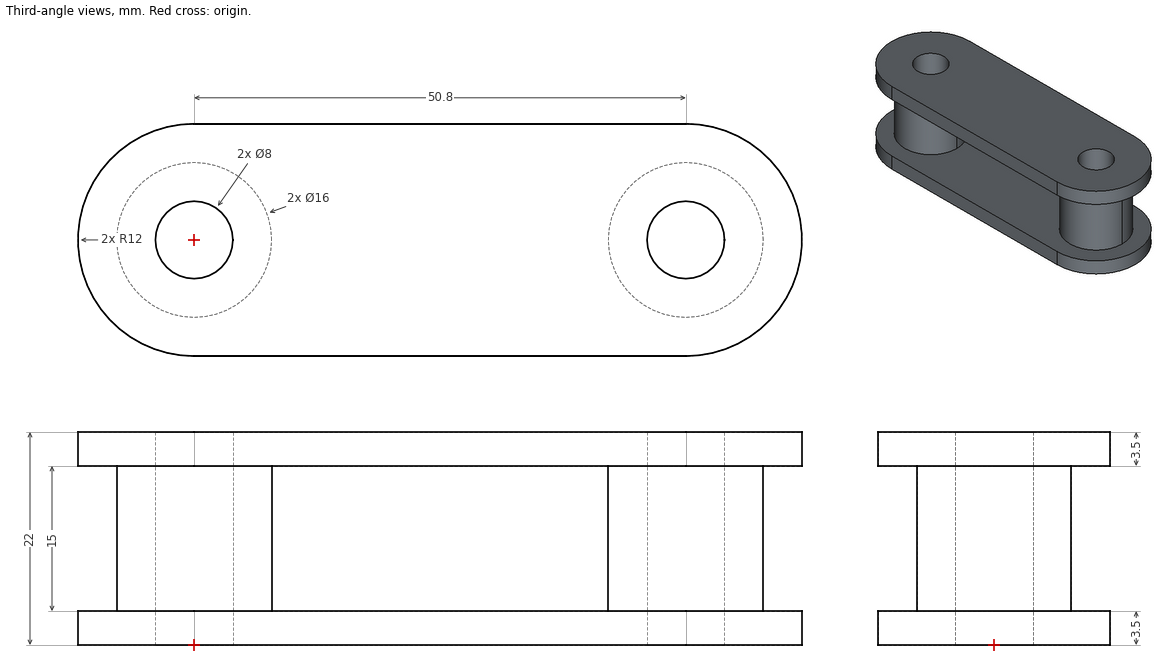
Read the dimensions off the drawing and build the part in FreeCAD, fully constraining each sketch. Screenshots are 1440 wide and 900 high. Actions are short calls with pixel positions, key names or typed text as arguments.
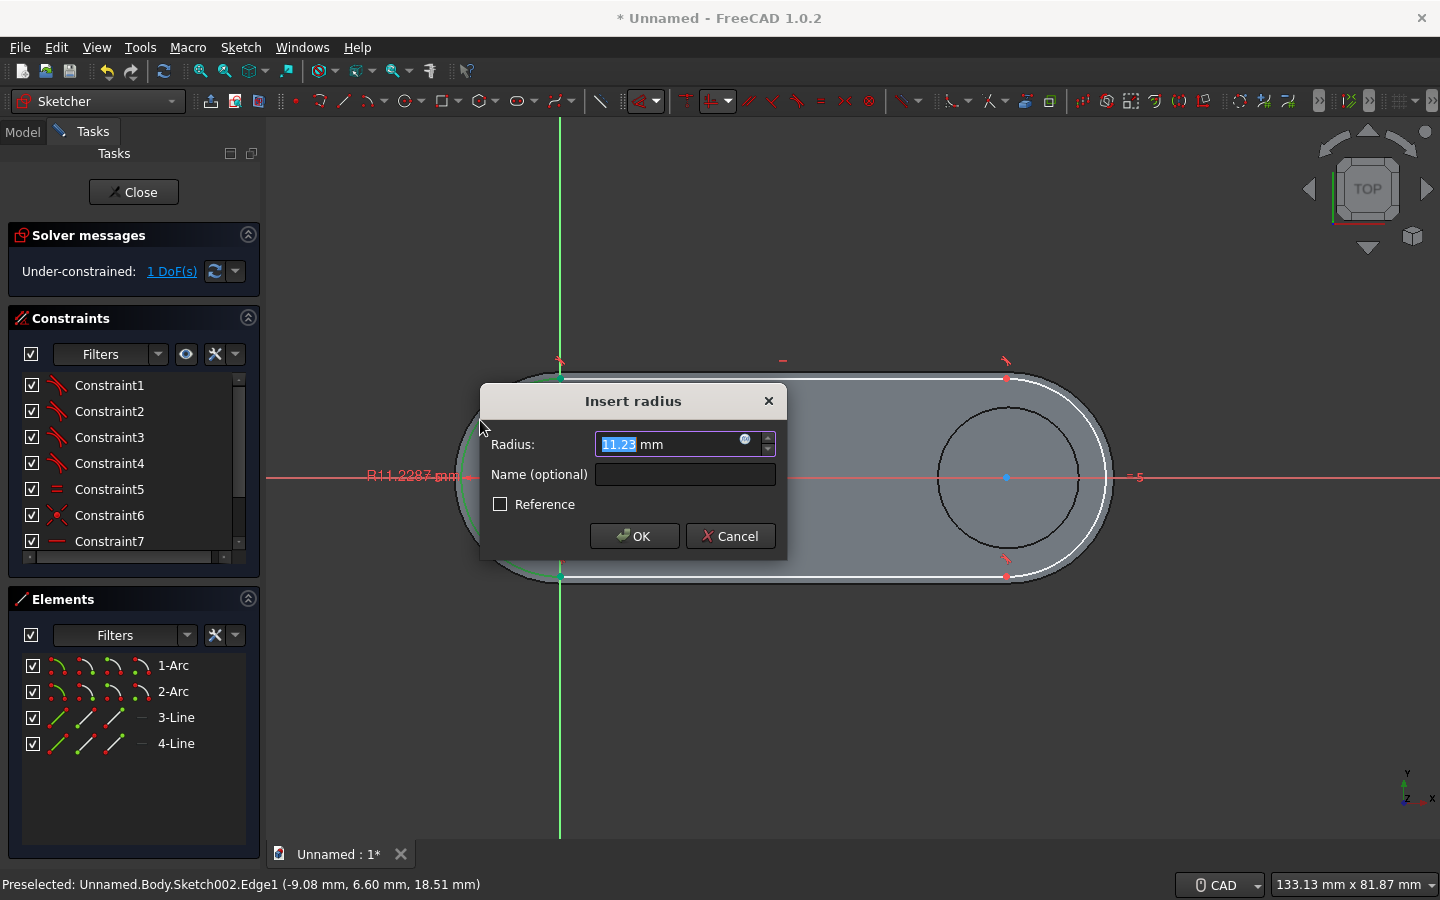
text(12)
key(Return)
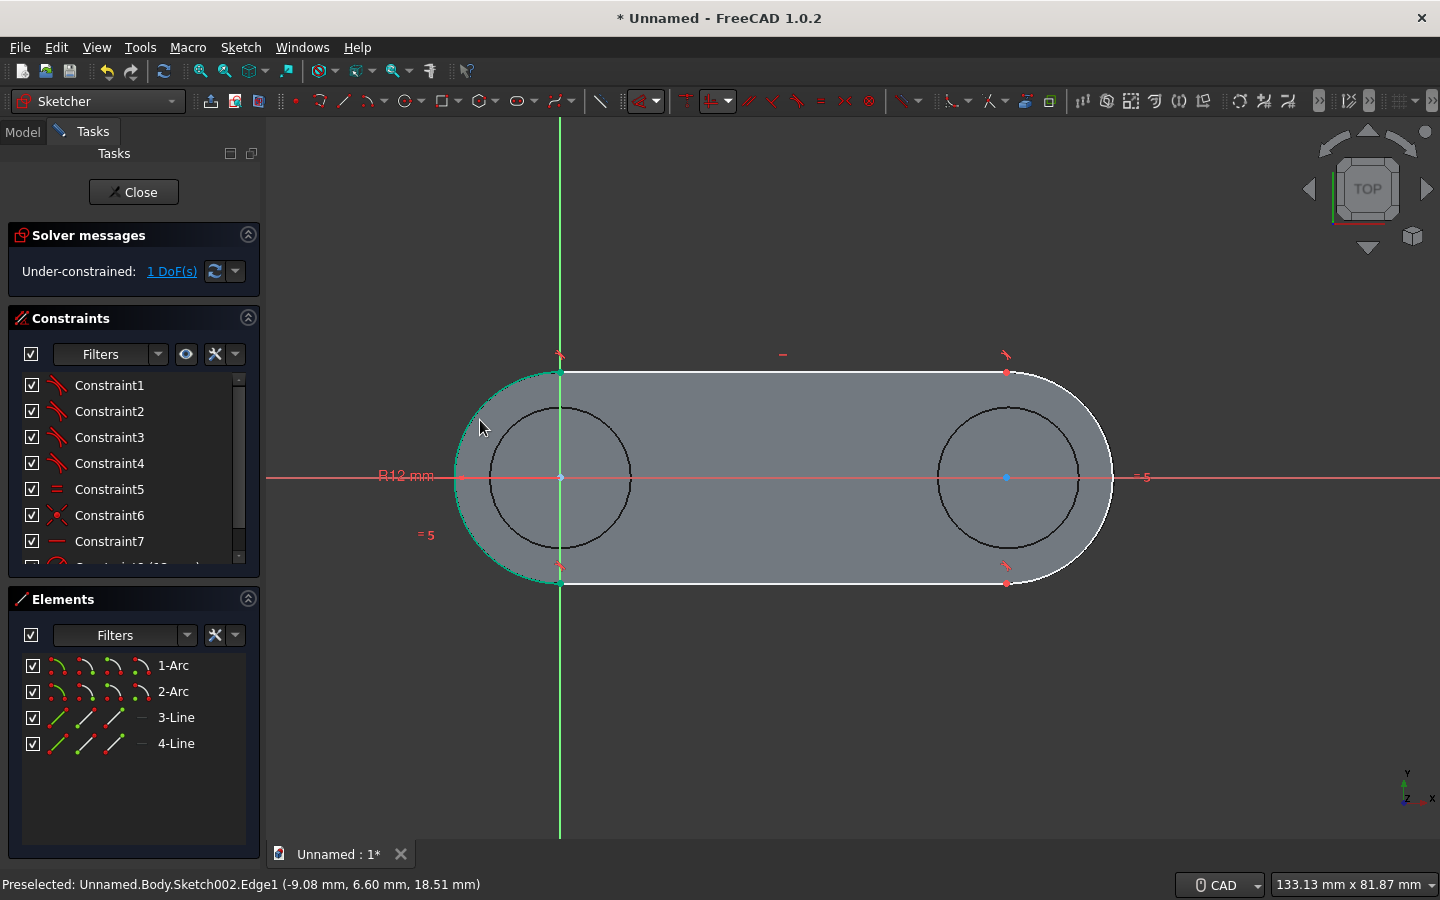
click(694, 372)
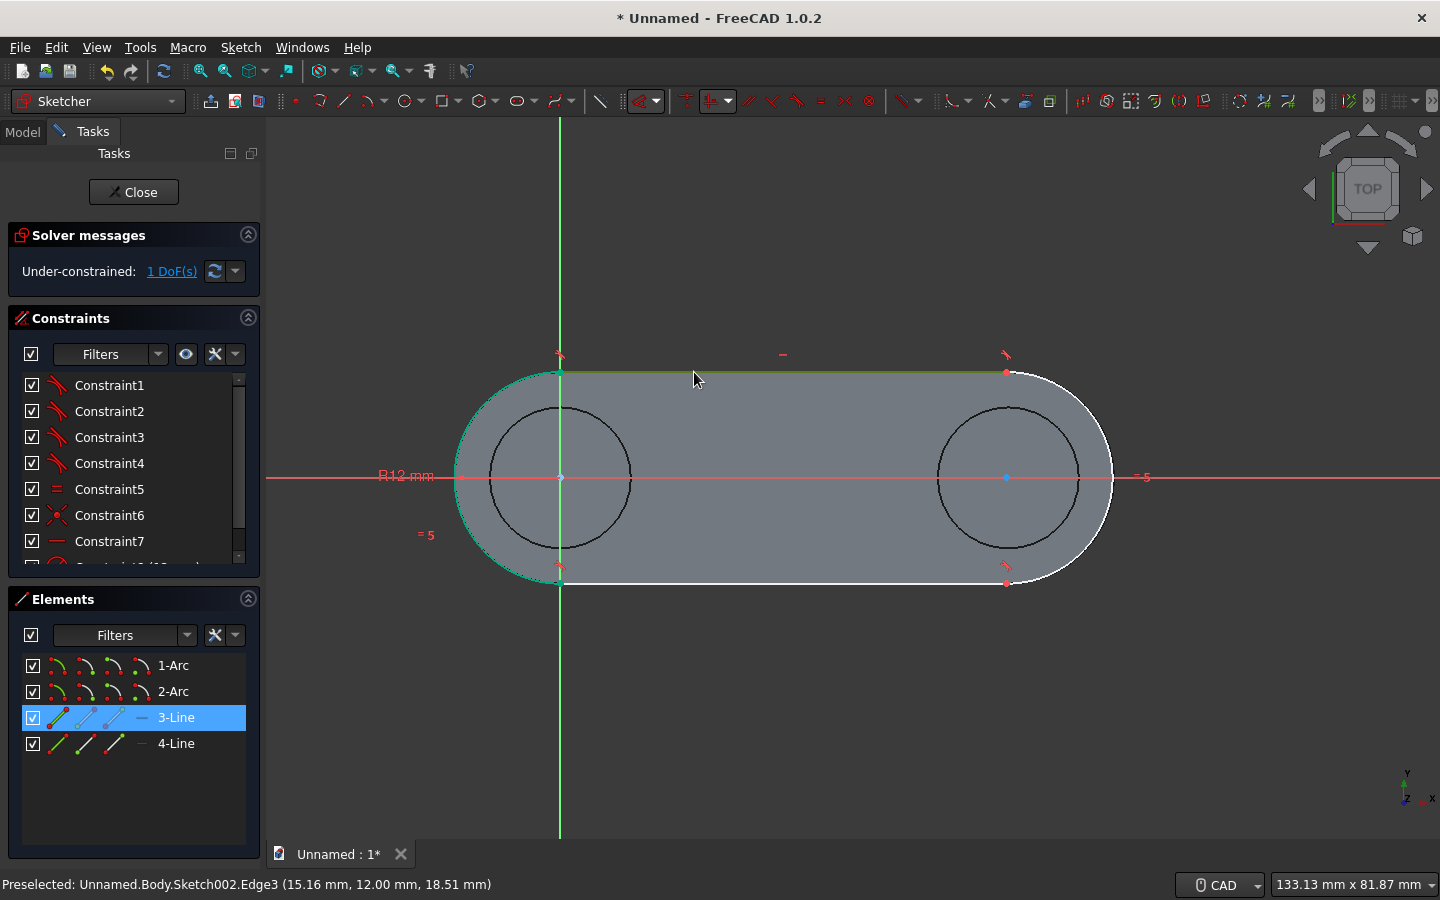
key(l)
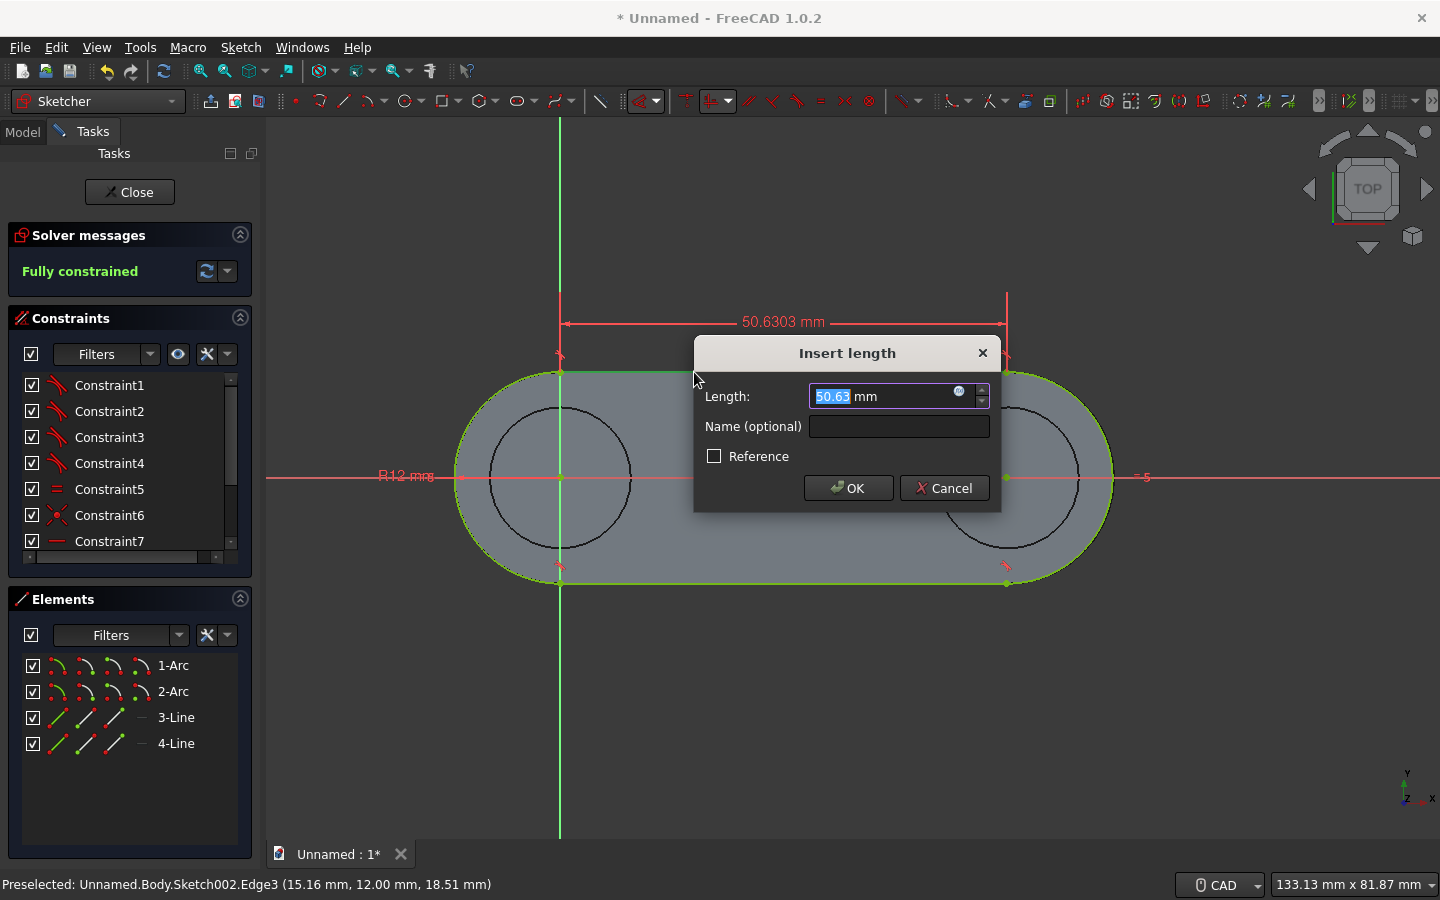
text(50.8)
key(Return)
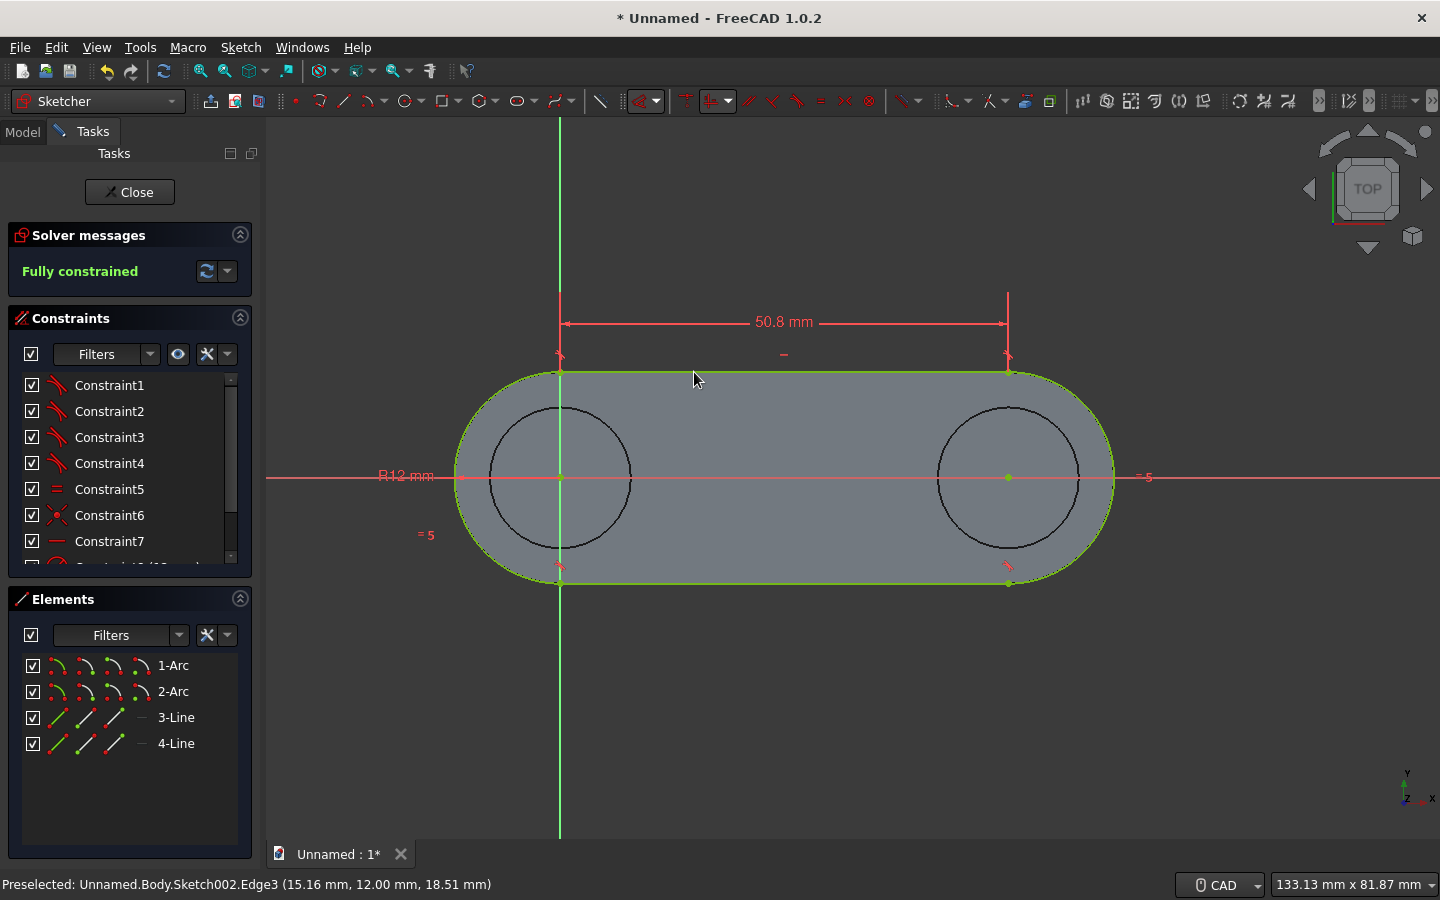
click(130, 192)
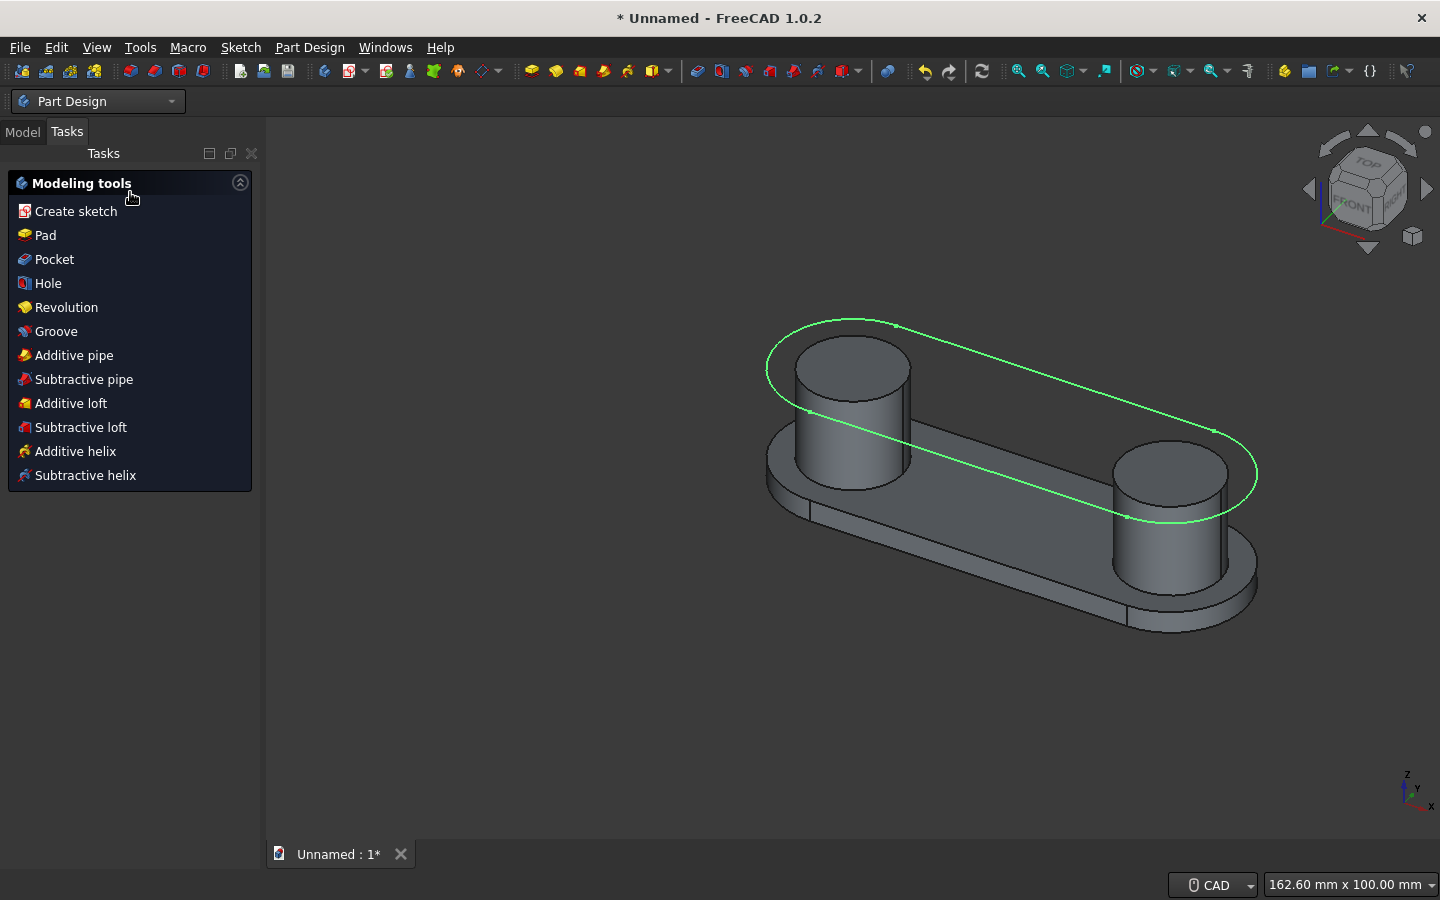
click(532, 72)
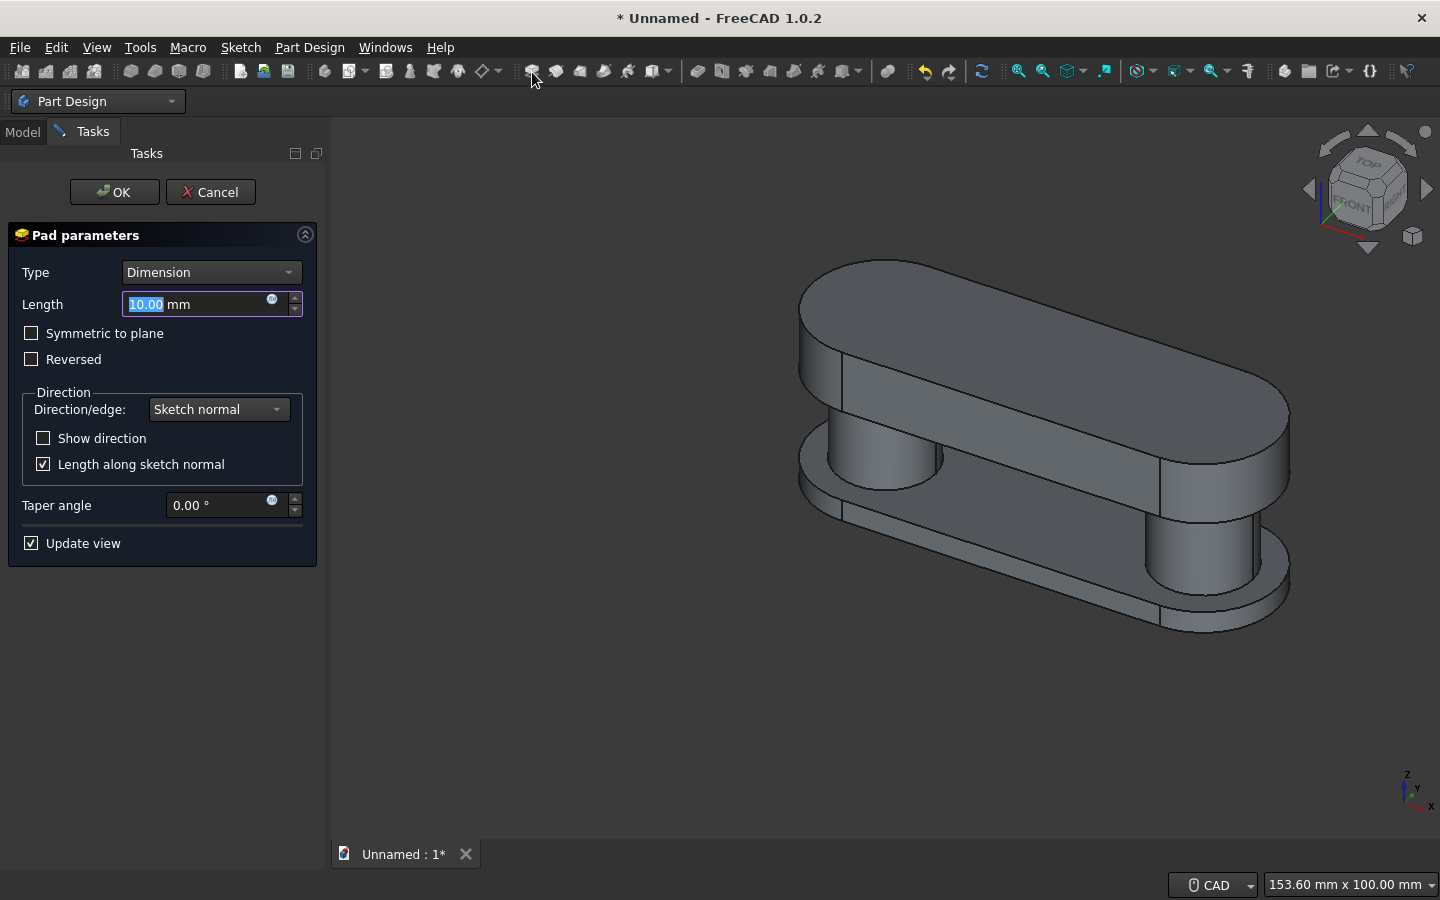
text(3.5)
key(Tab)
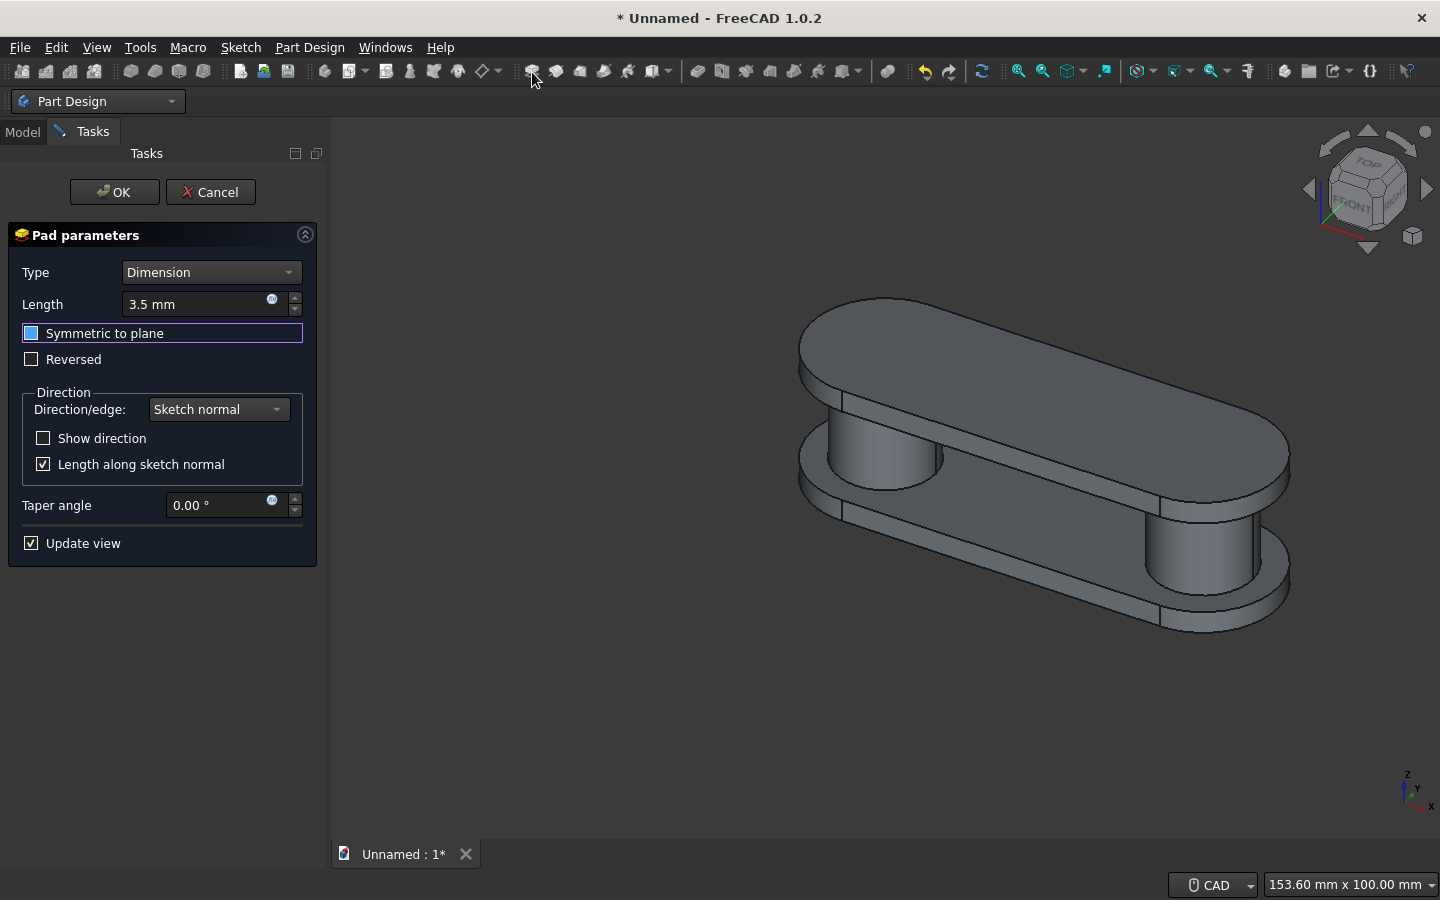
click(115, 192)